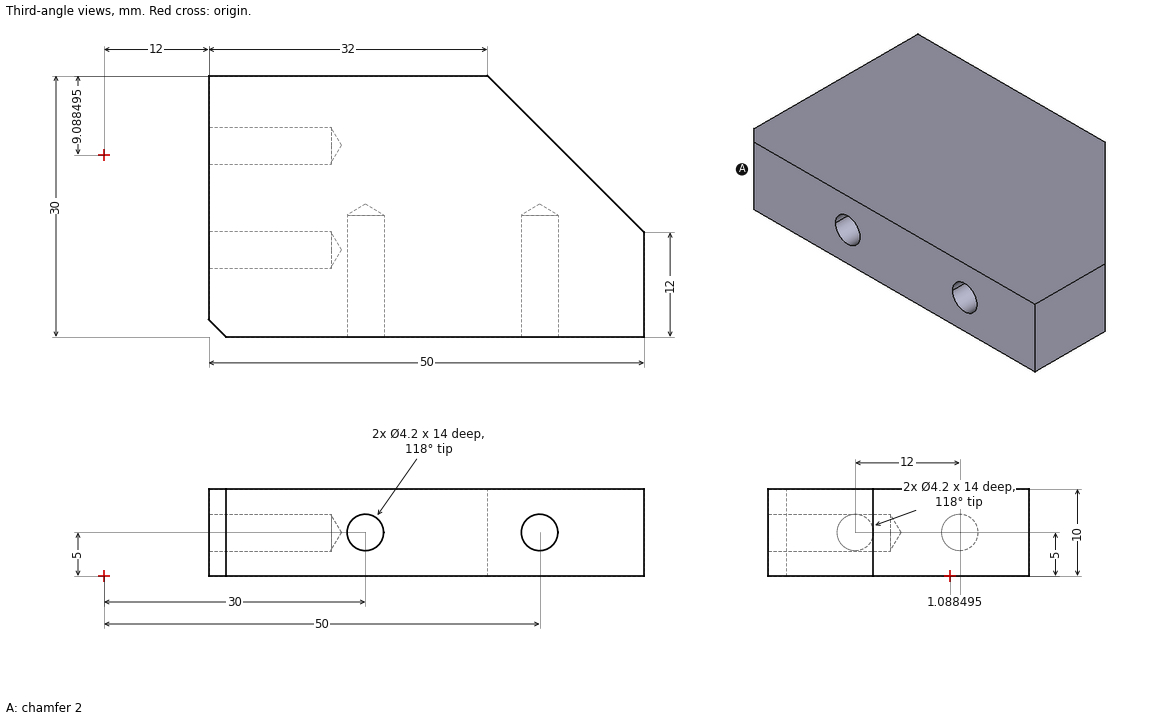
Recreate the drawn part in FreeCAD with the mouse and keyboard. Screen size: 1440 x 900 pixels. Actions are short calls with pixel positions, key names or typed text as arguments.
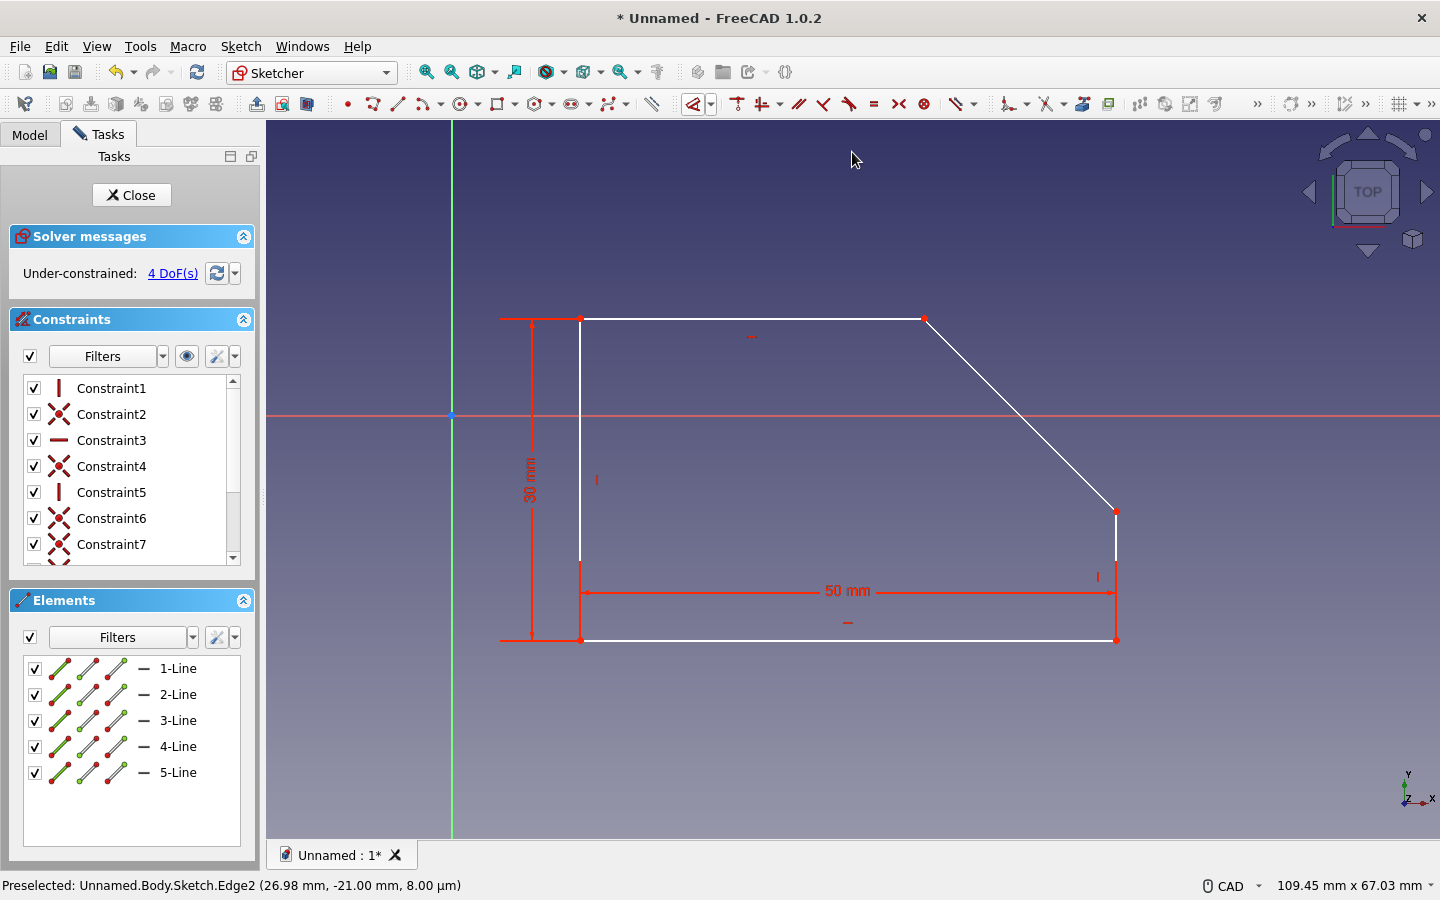
click(1116, 602)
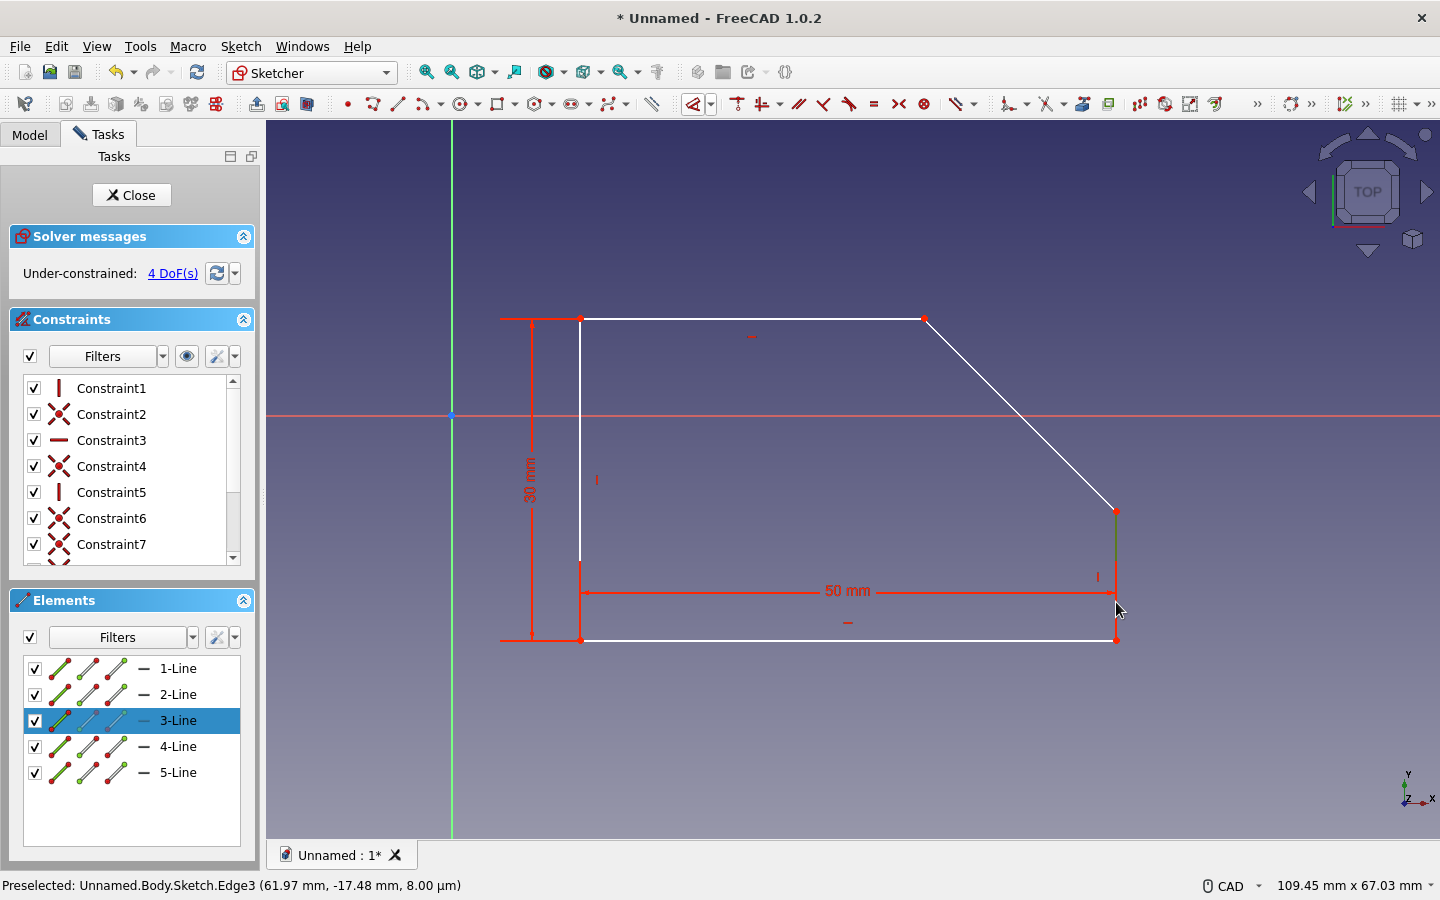
click(710, 104)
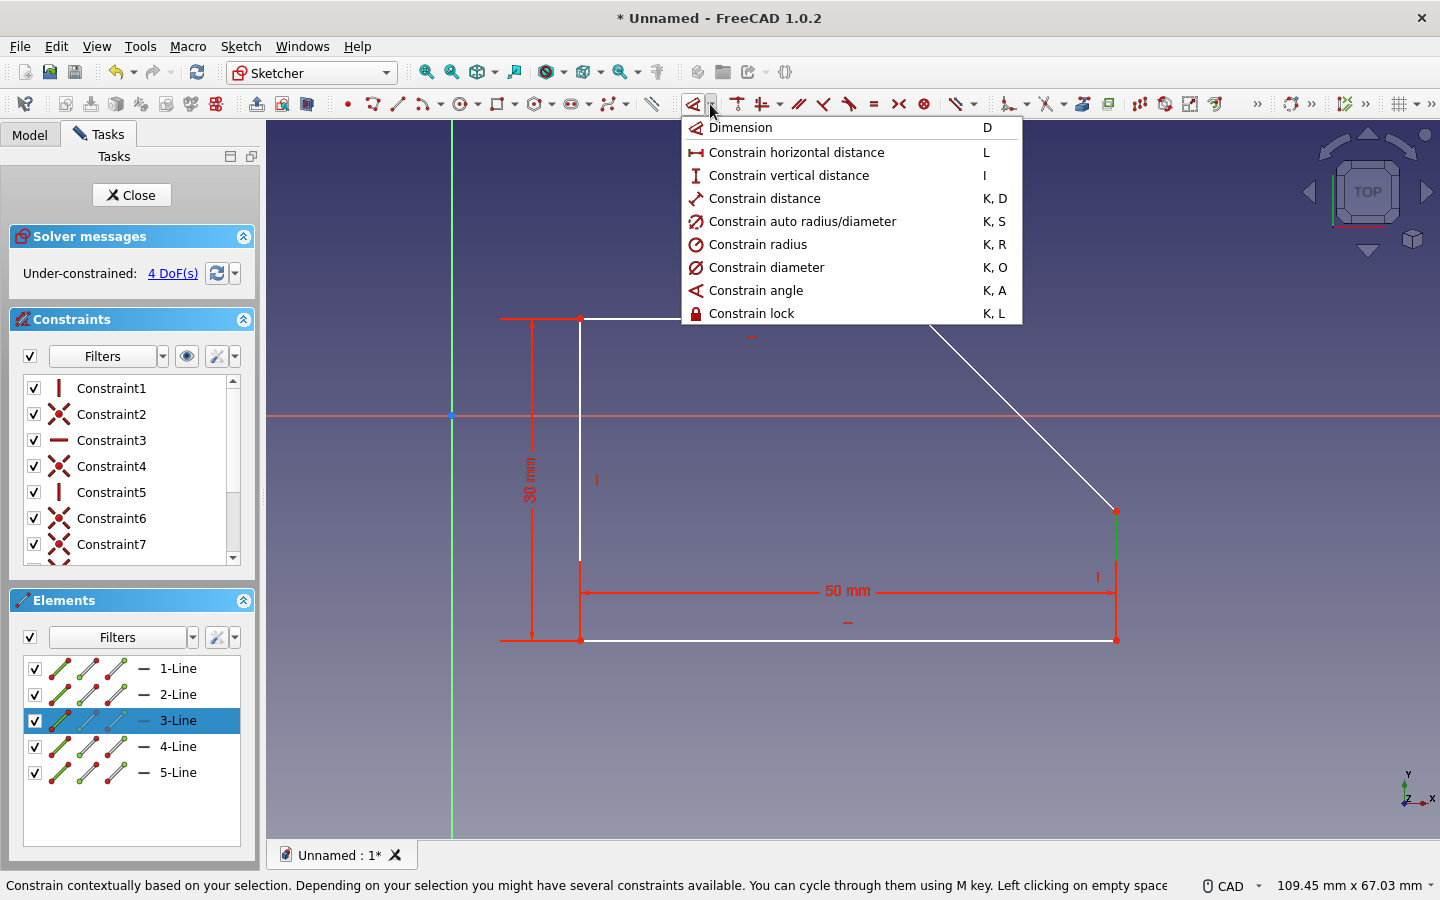
click(852, 176)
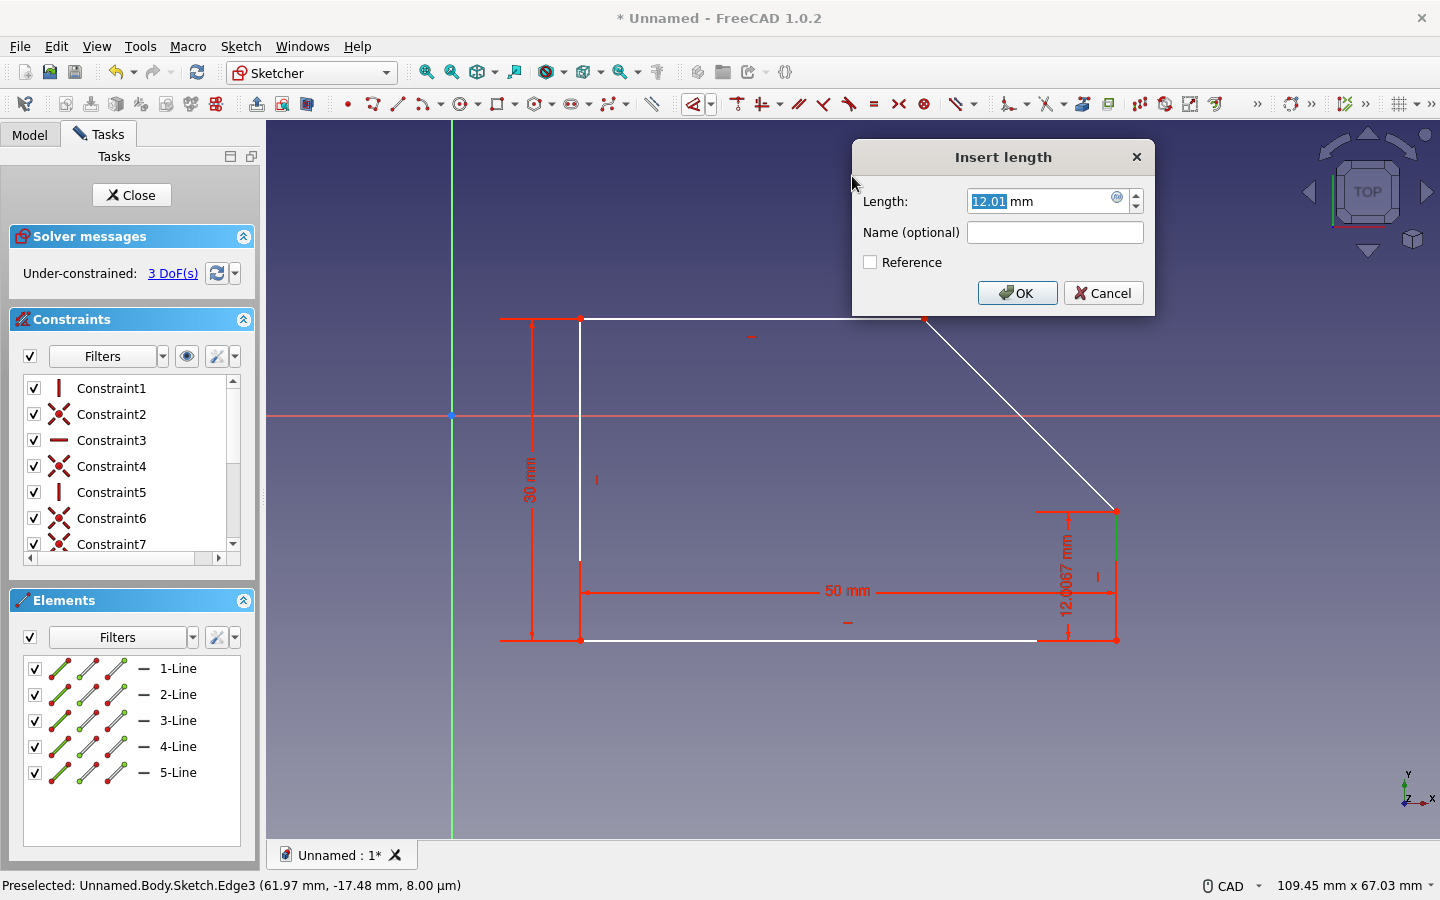
text(12)
key(Return)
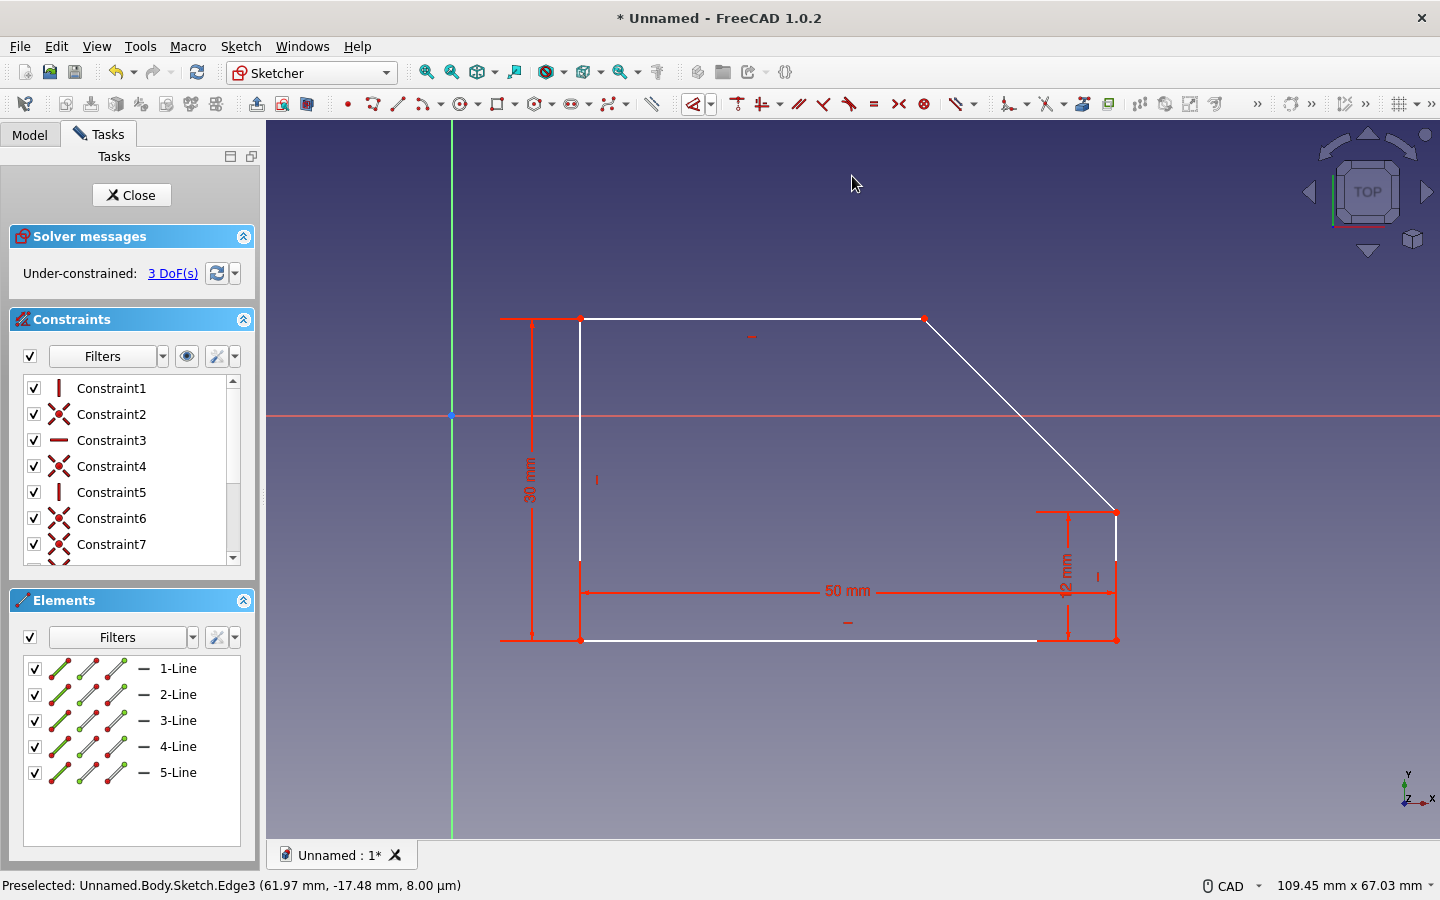
click(821, 319)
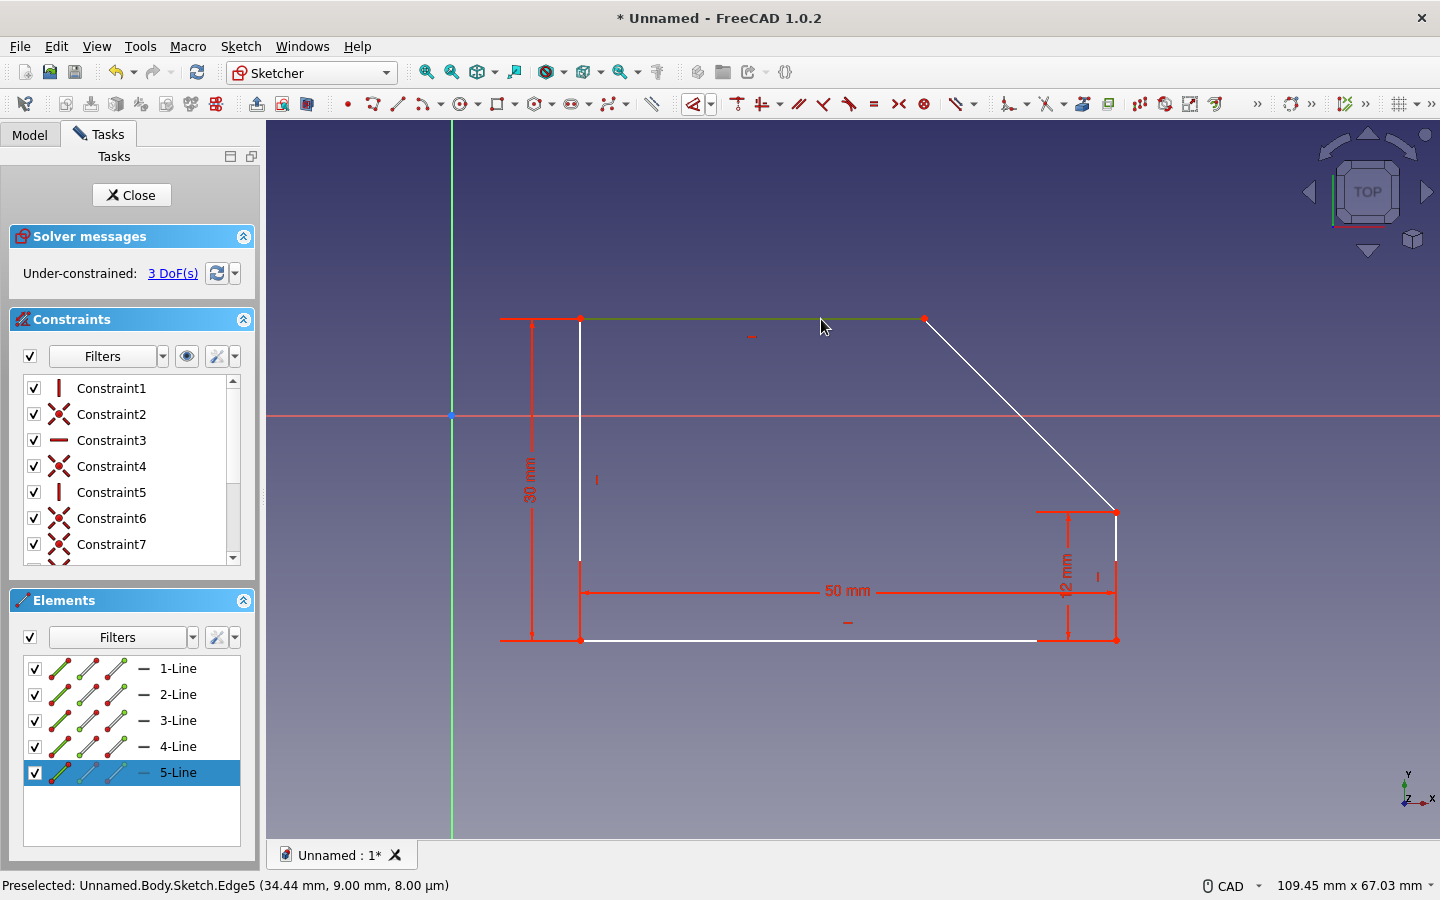
click(710, 104)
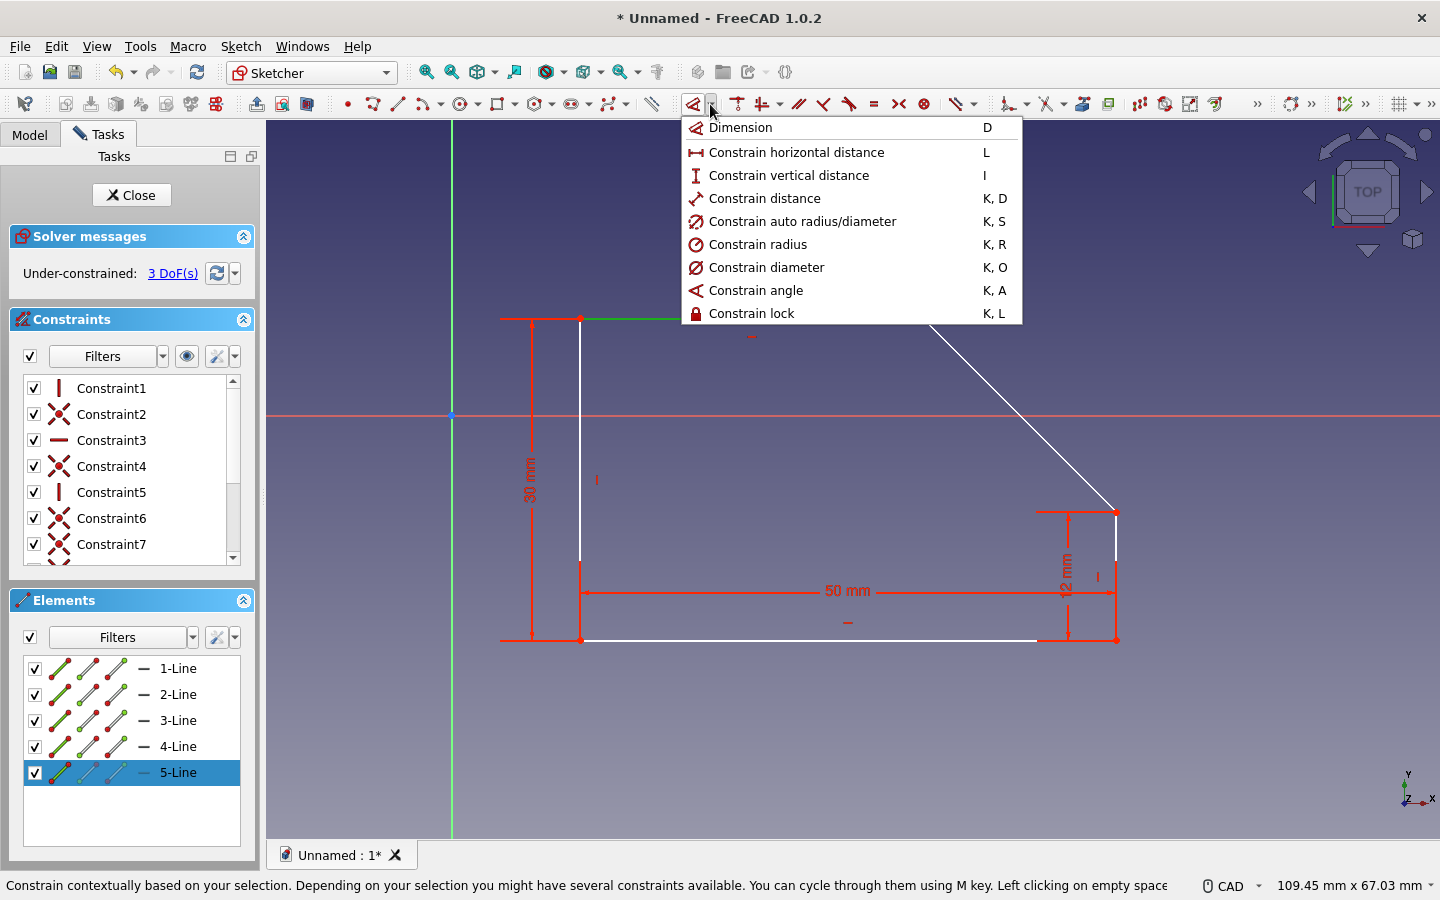
click(852, 152)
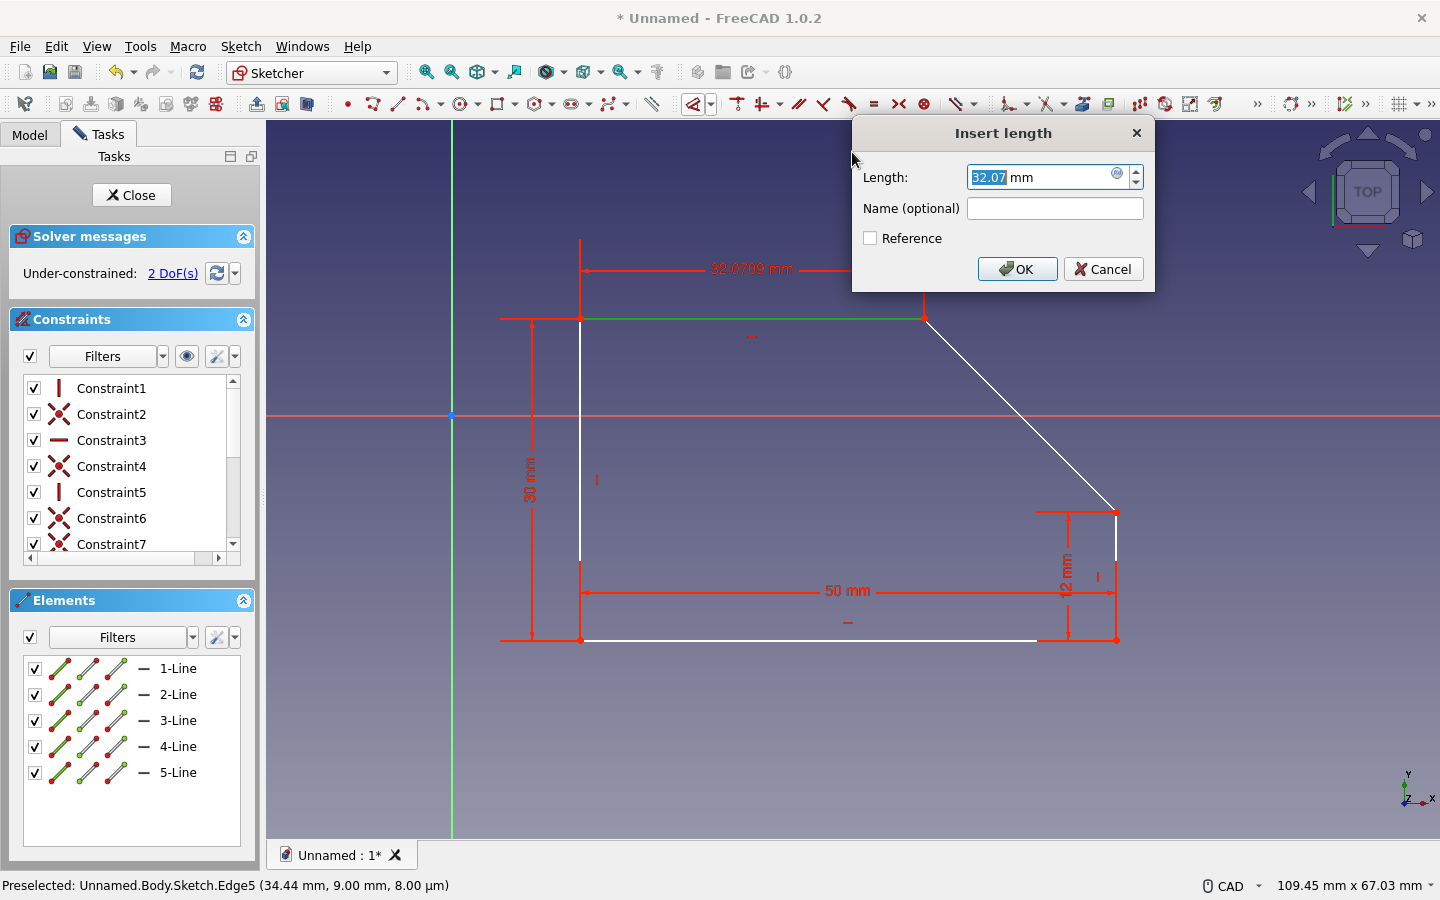
text(32)
key(Return)